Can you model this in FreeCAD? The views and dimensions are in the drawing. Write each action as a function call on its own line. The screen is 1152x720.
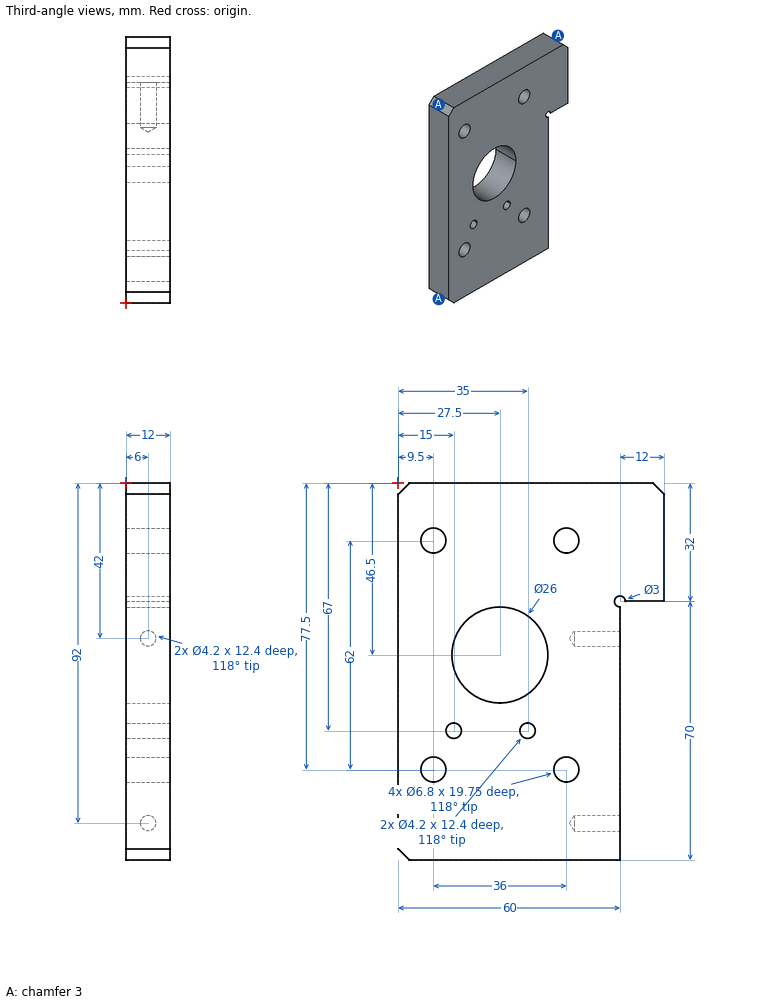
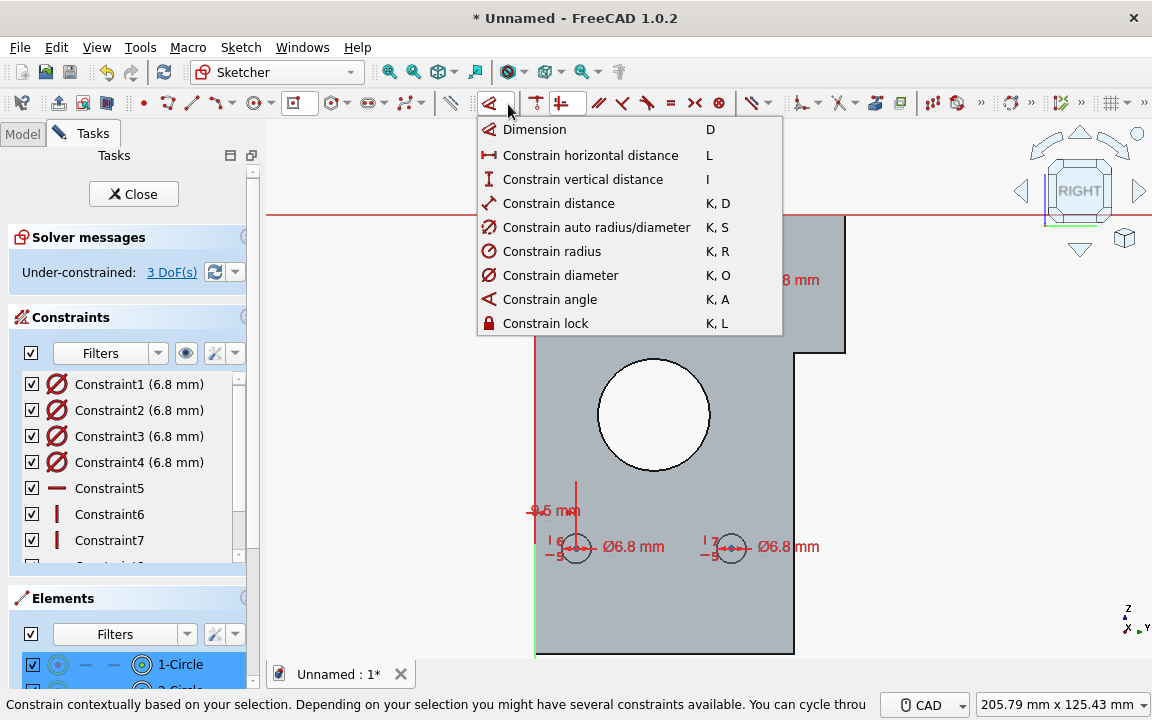
click(630, 155)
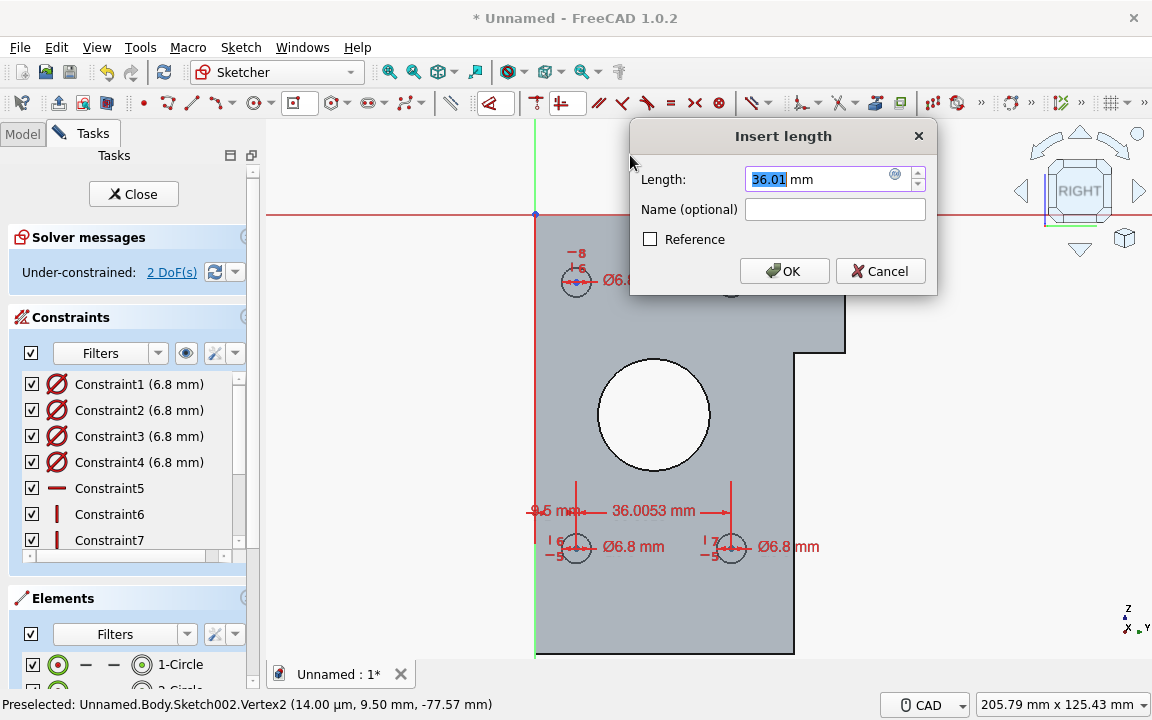
text(36)
key(Return)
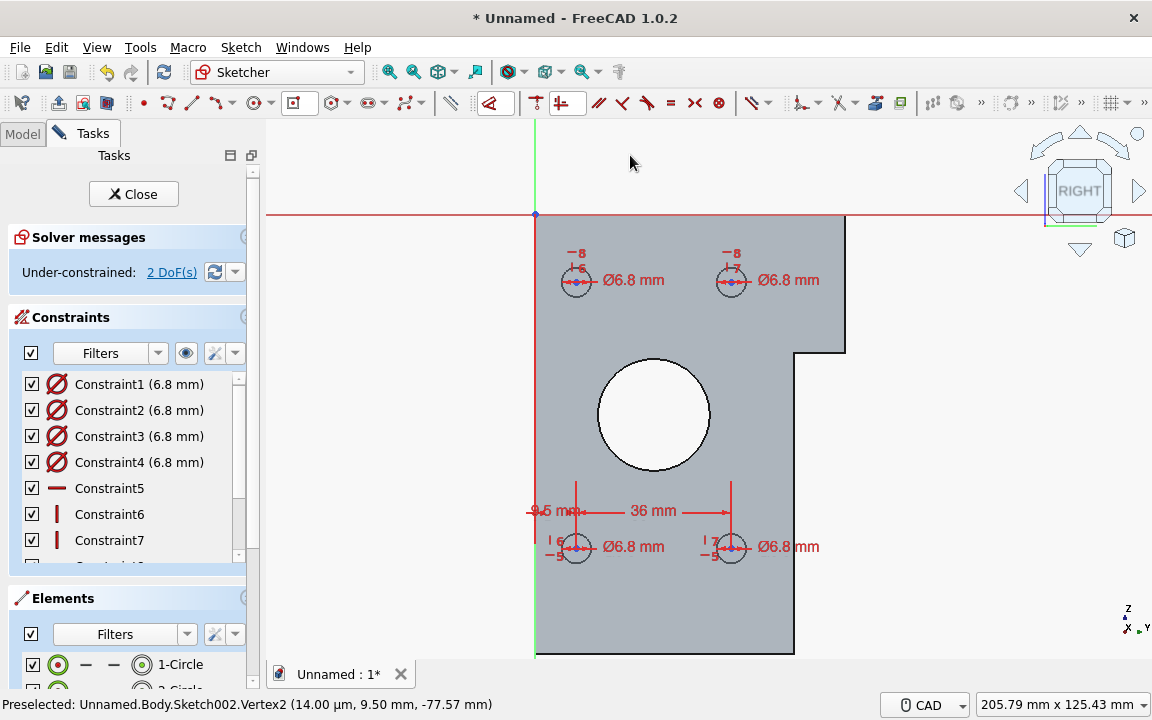
click(576, 549)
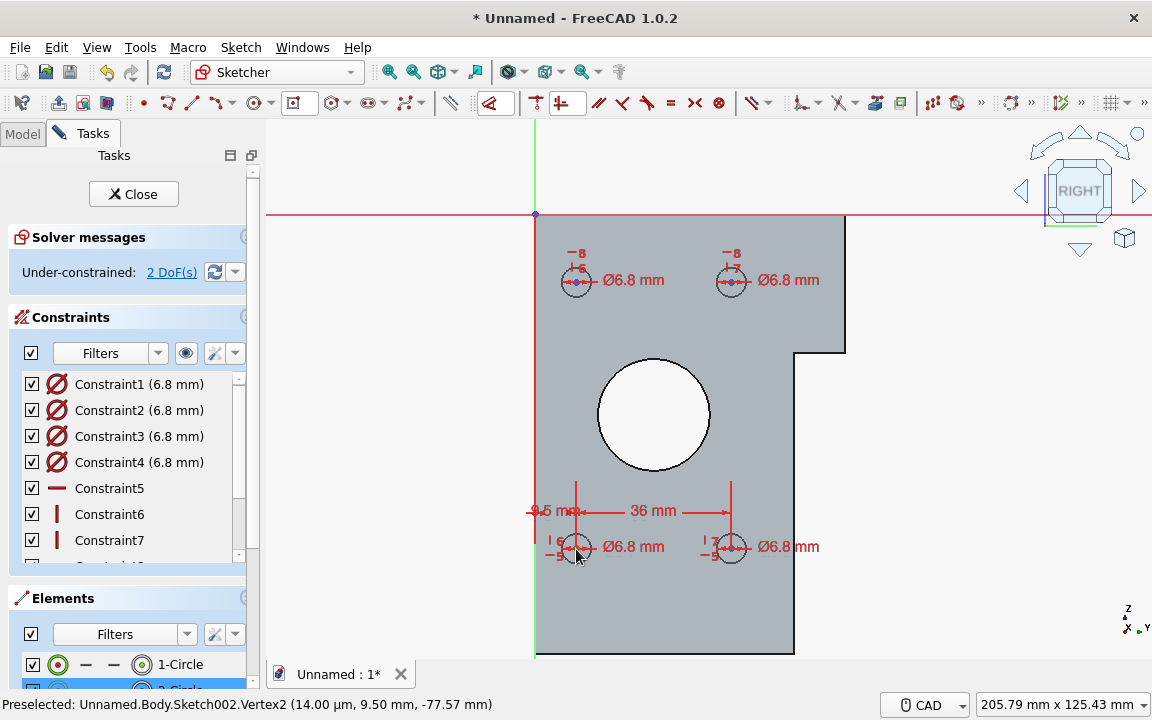
click(576, 282)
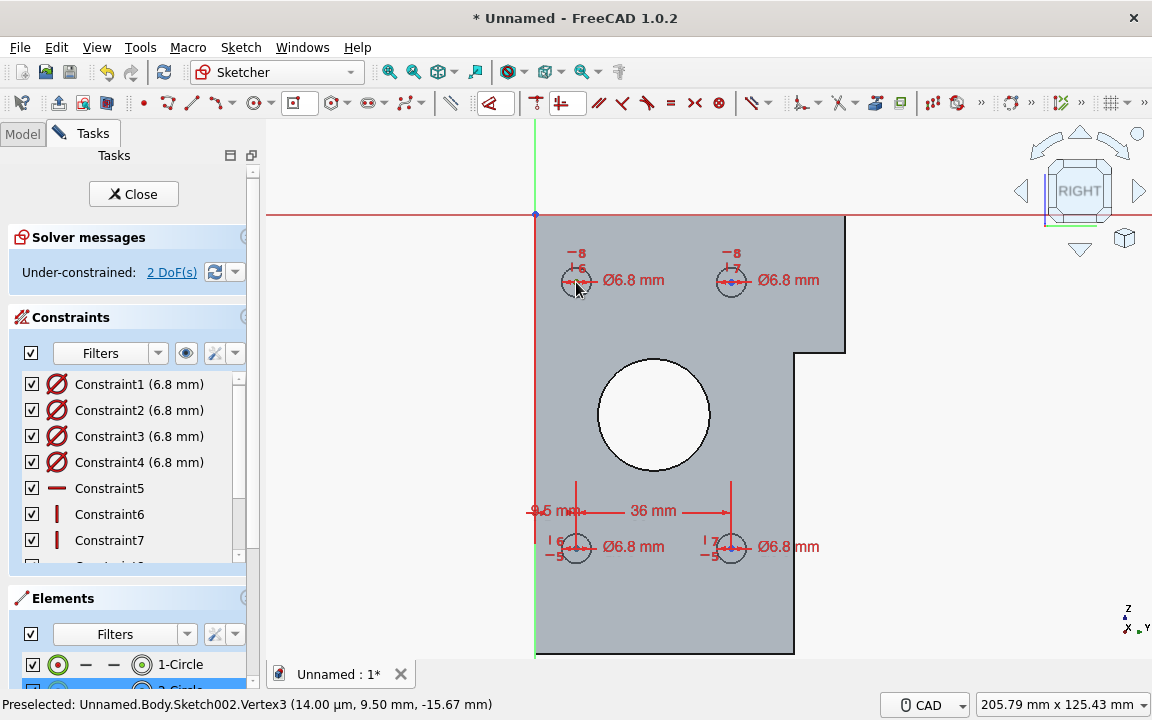
key(i)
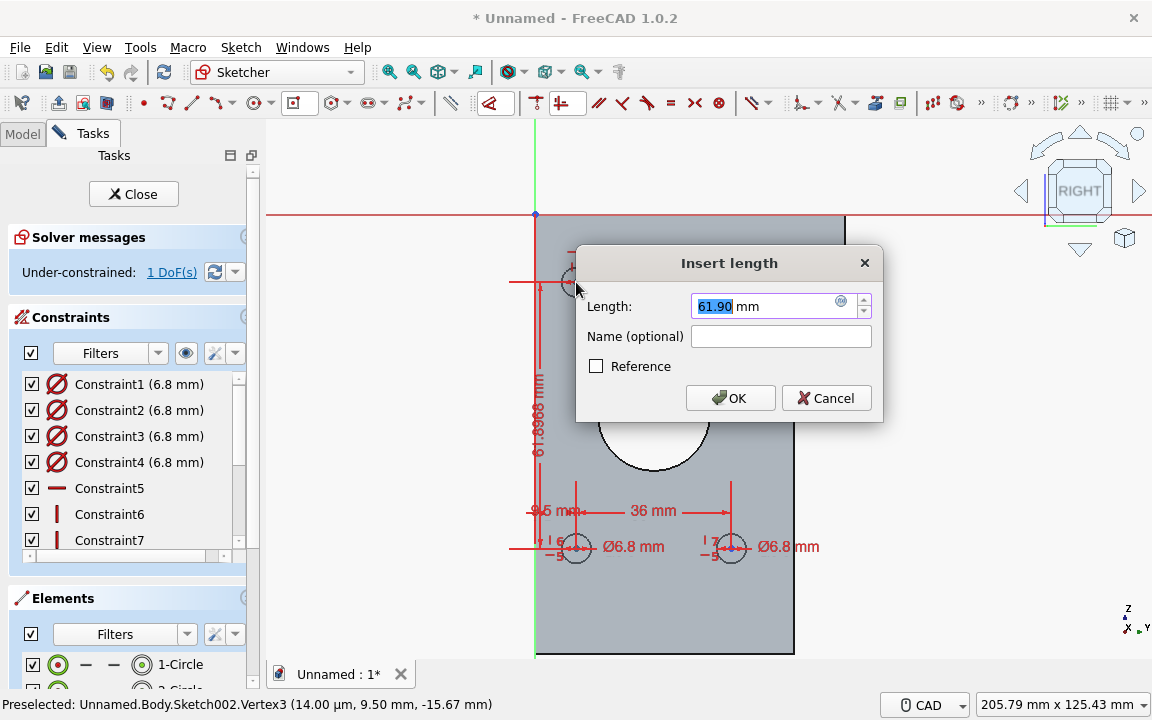
text(62)
key(Return)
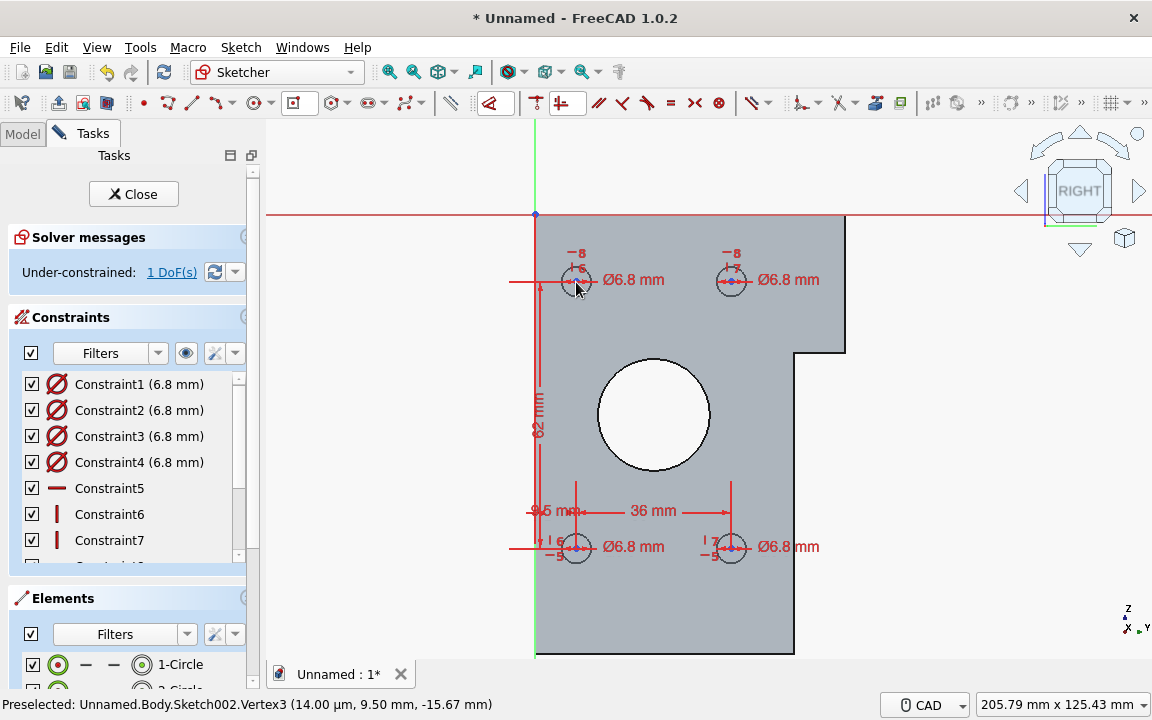
click(731, 549)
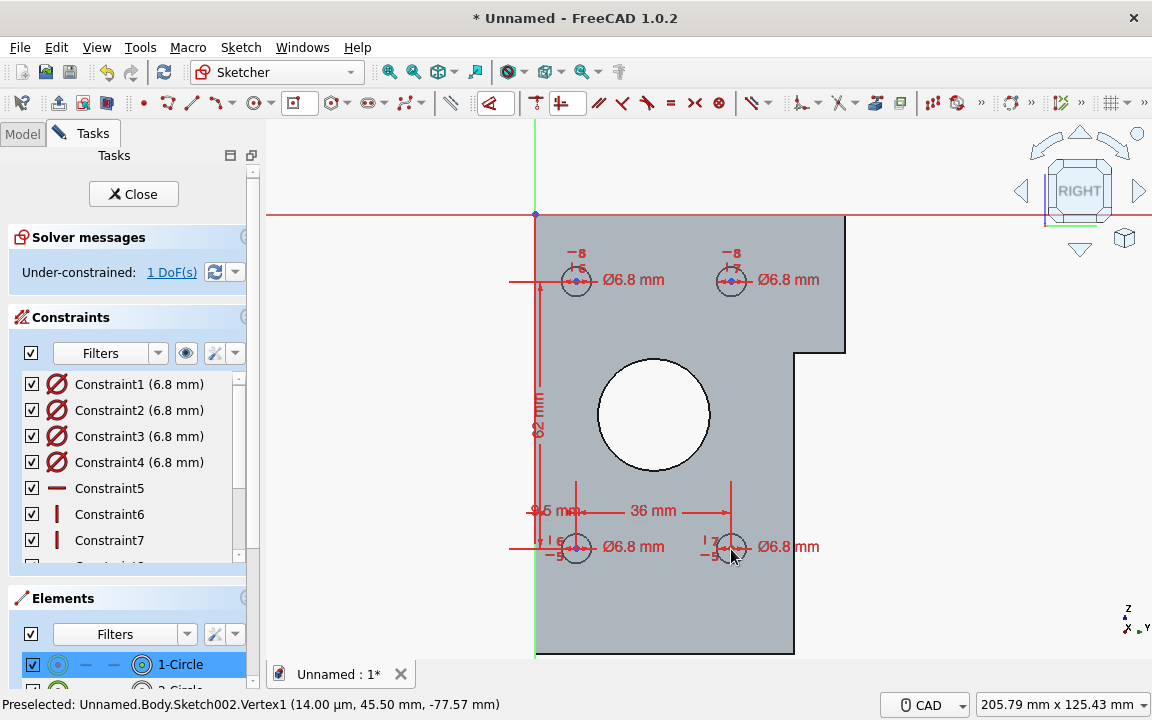
key(i)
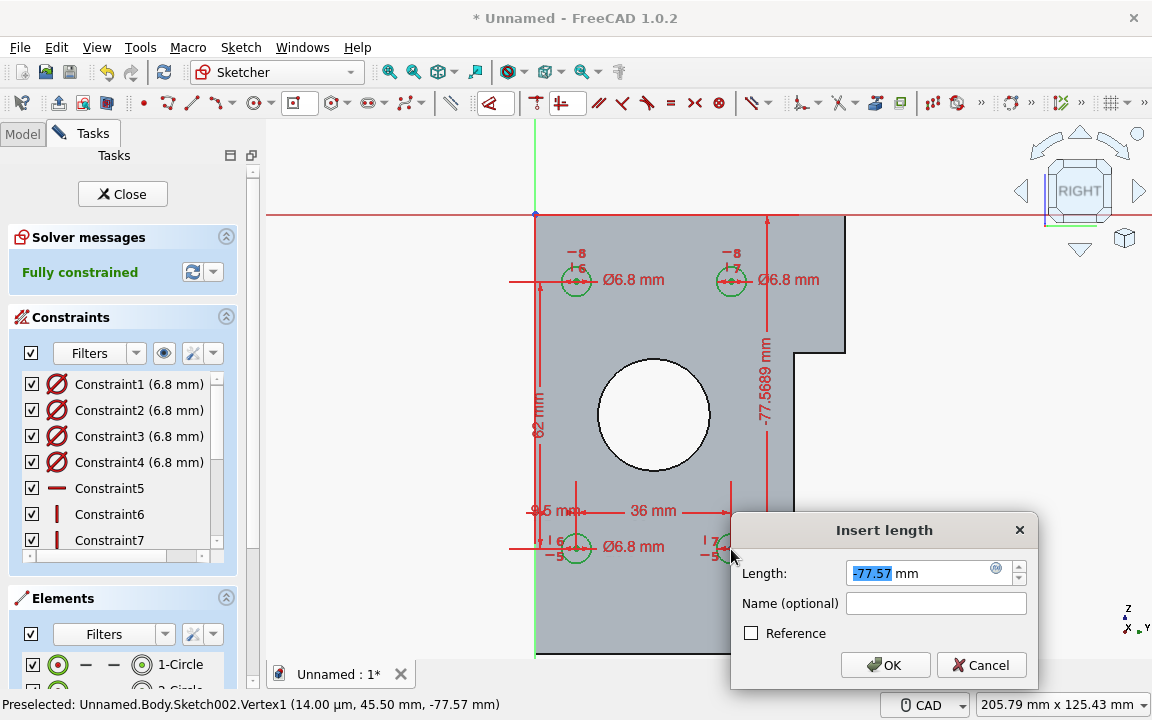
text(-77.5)
key(Return)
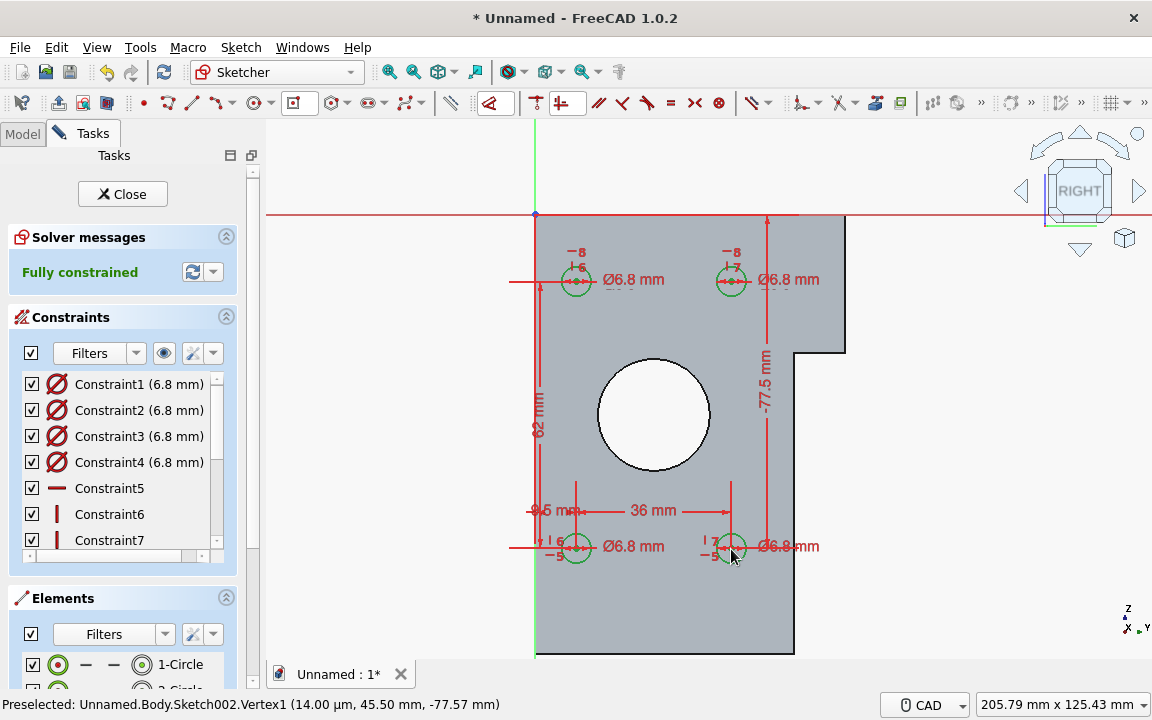
click(123, 194)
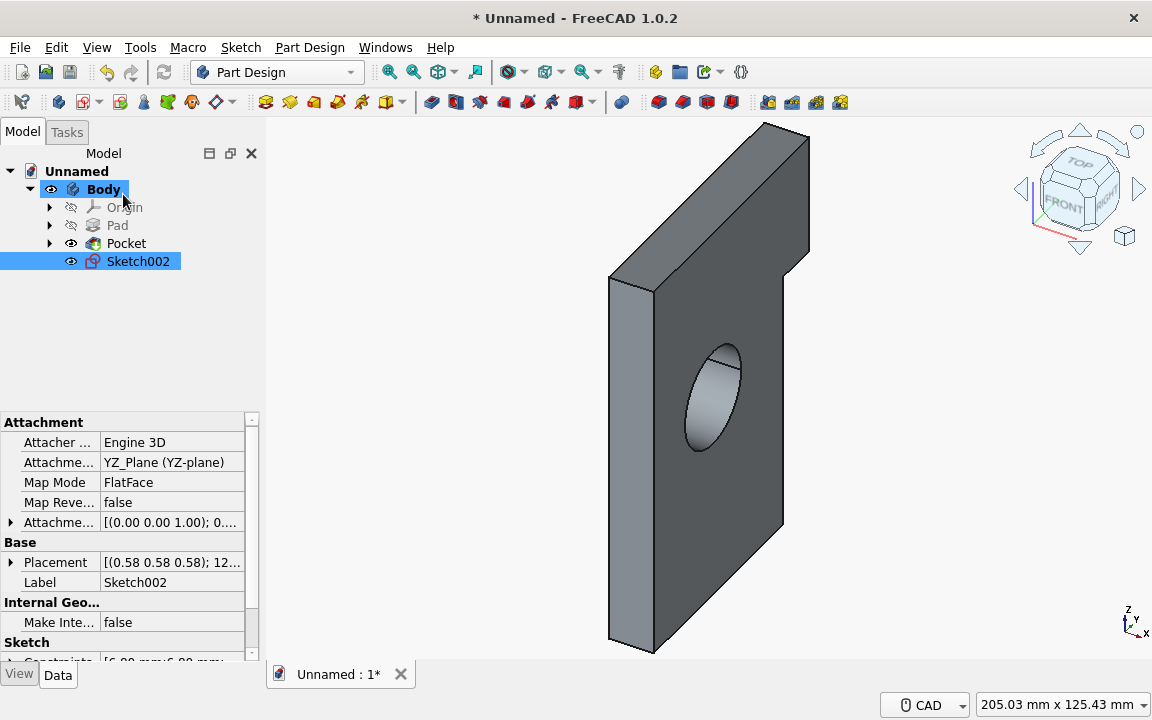
click(456, 102)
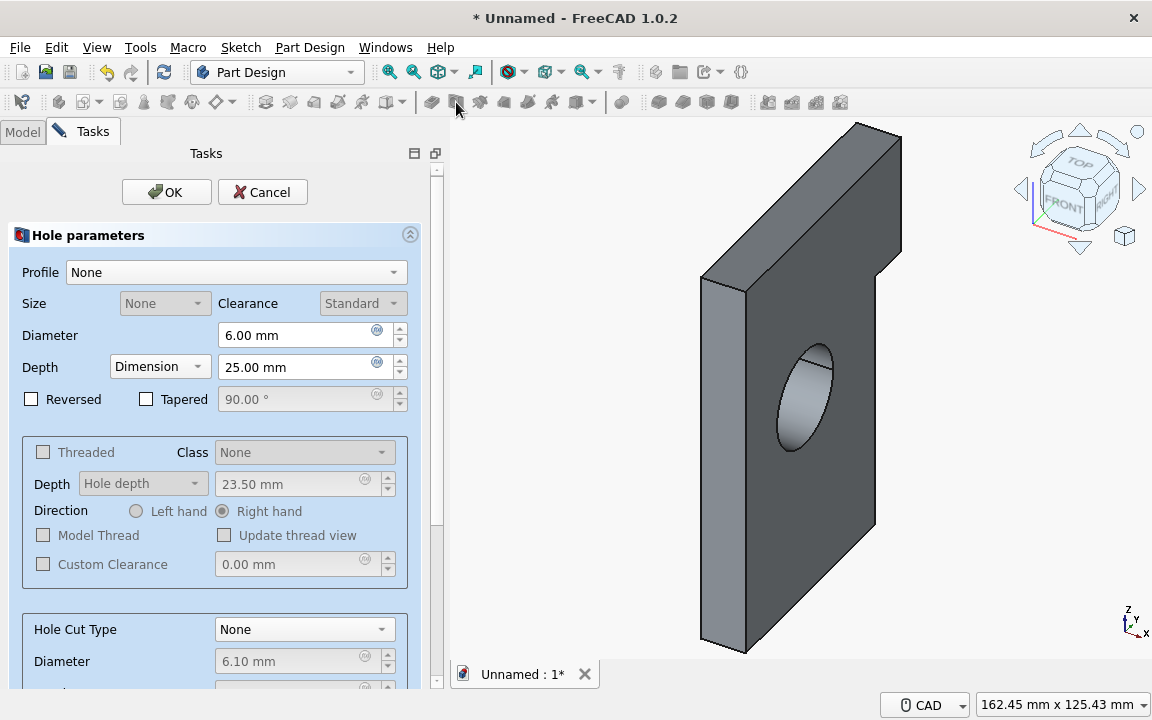
triple_click(305, 335)